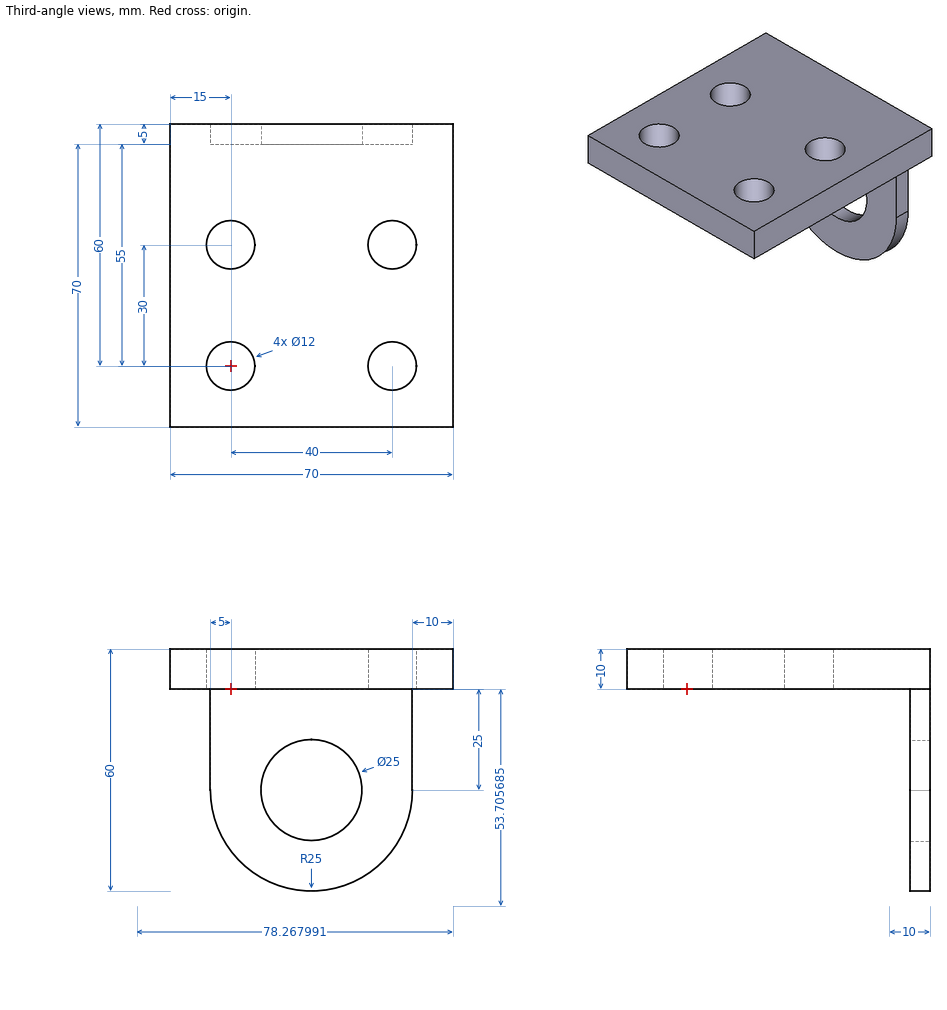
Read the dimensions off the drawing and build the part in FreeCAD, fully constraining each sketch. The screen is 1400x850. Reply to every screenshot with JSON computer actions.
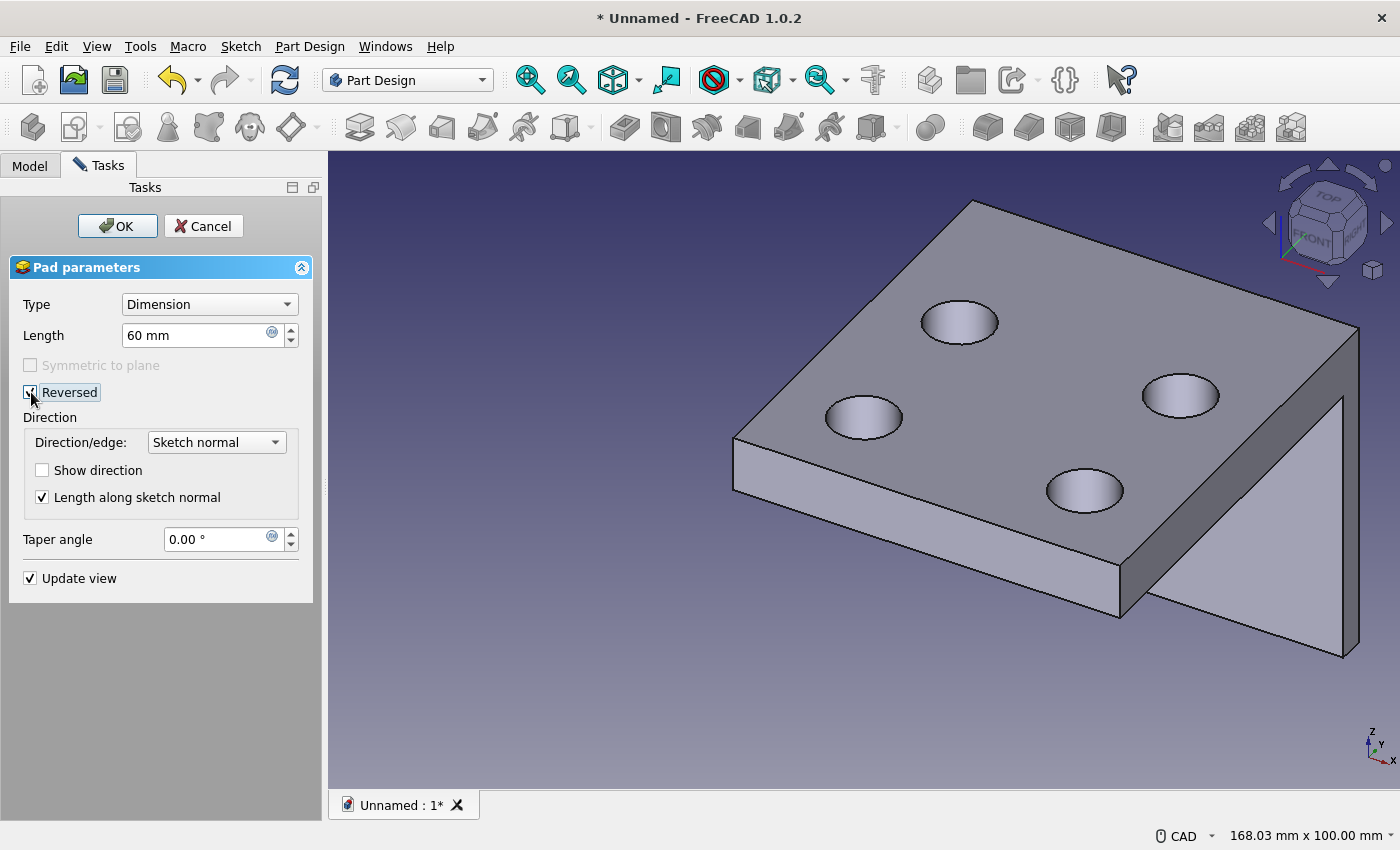
{"action": "left_click", "coordinate": [118, 226]}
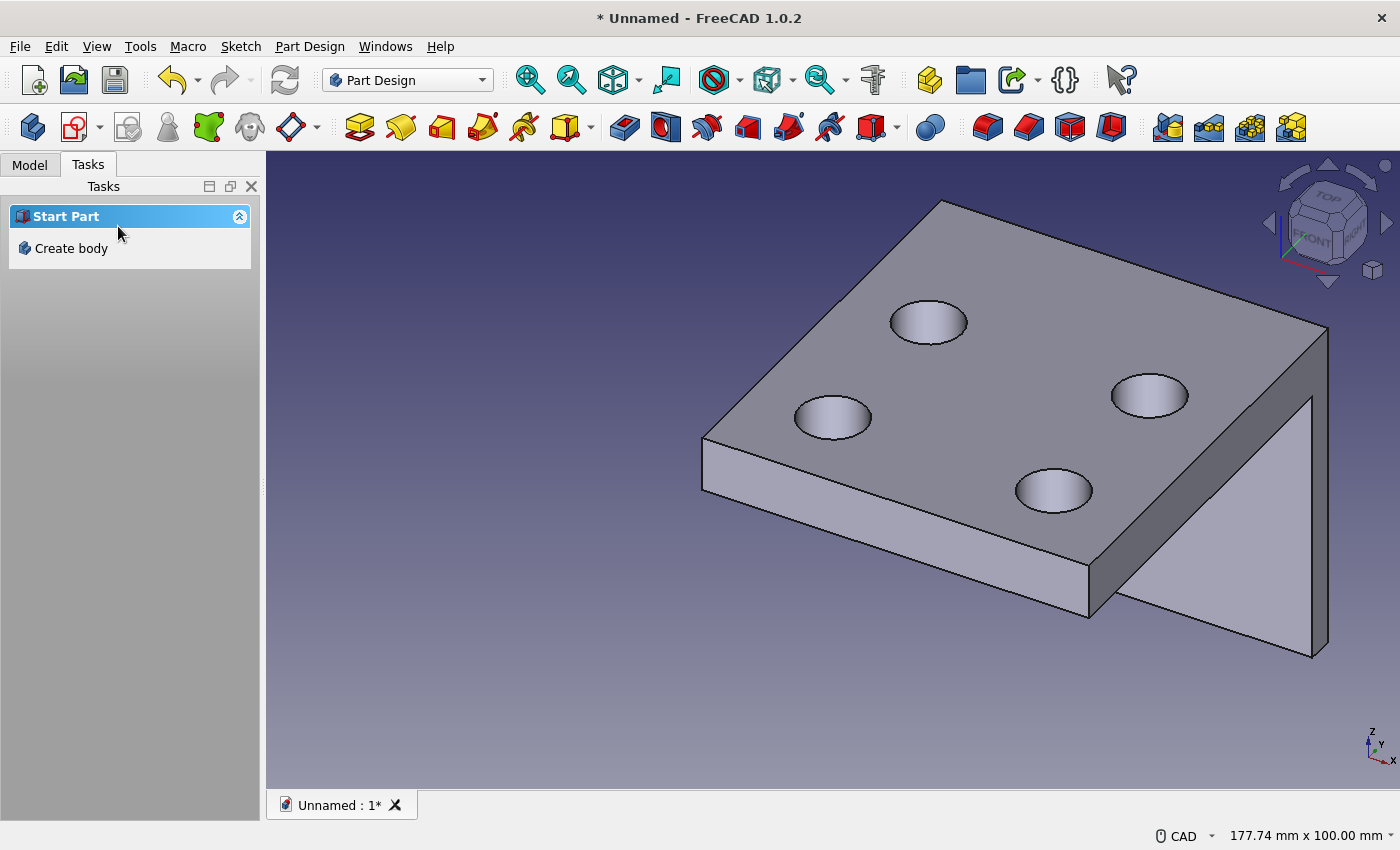
{"action": "left_click", "coordinate": [531, 80]}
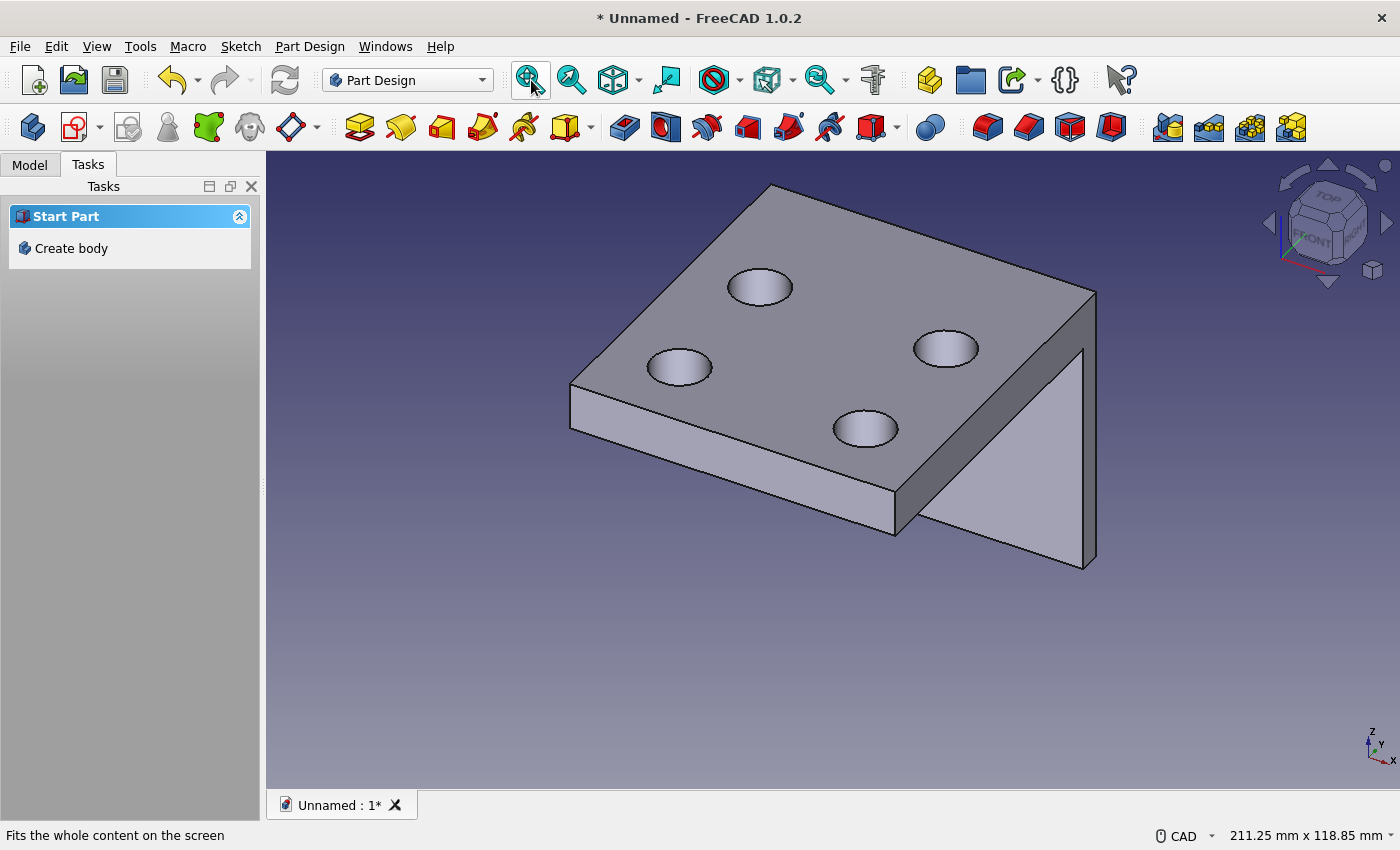
{"action": "key", "text": "4"}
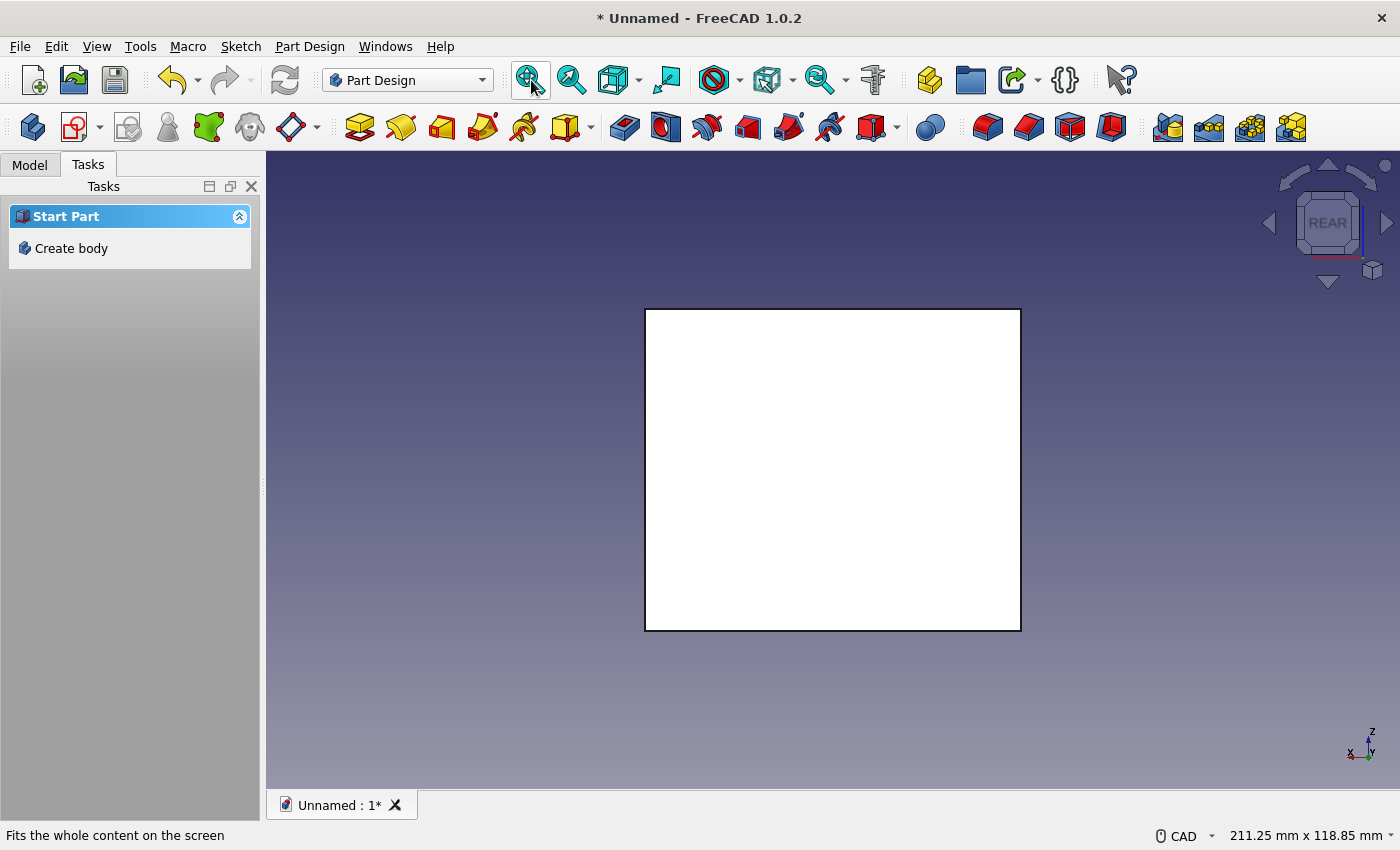
{"action": "left_click", "coordinate": [833, 469]}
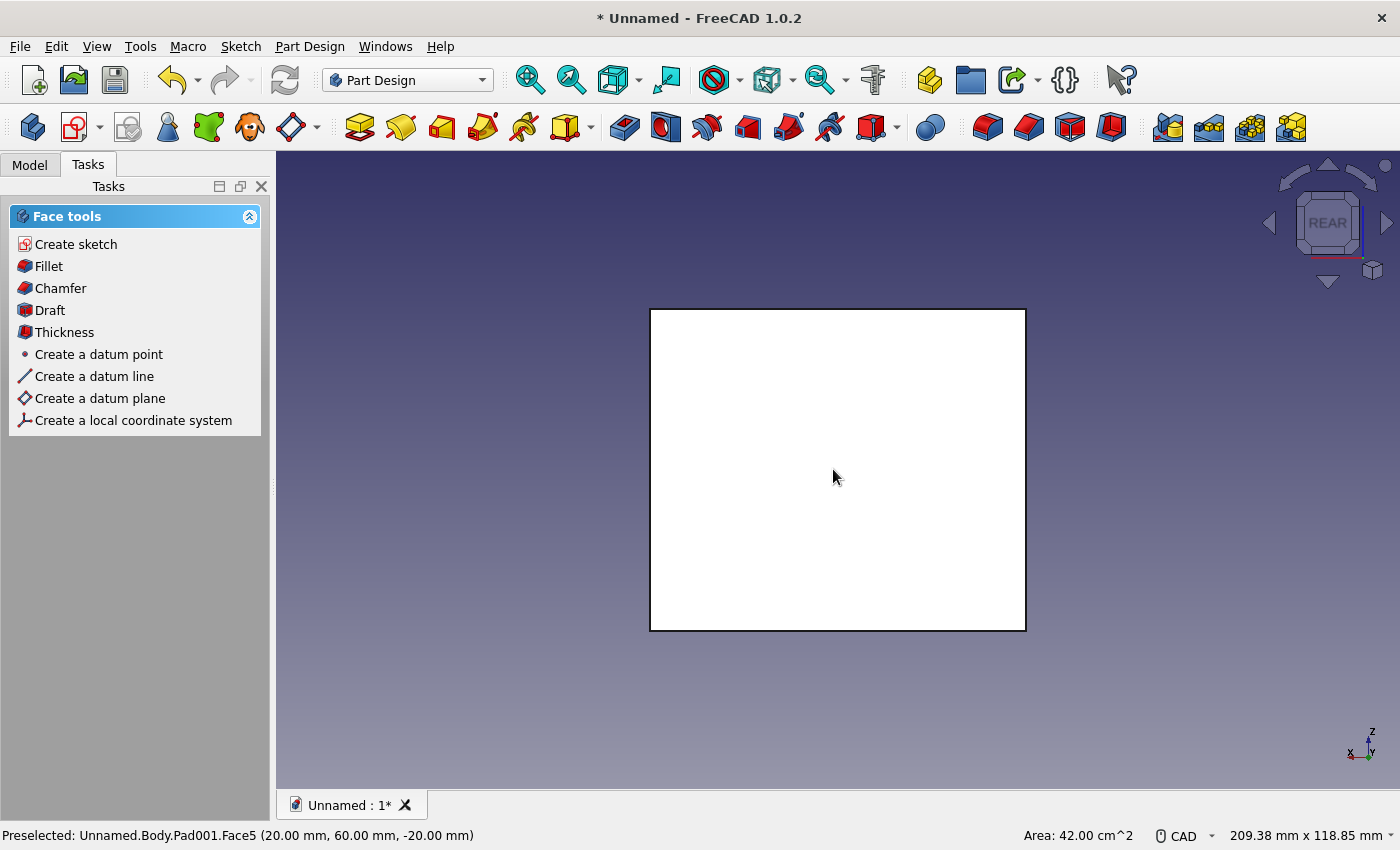
{"action": "left_click", "coordinate": [74, 128]}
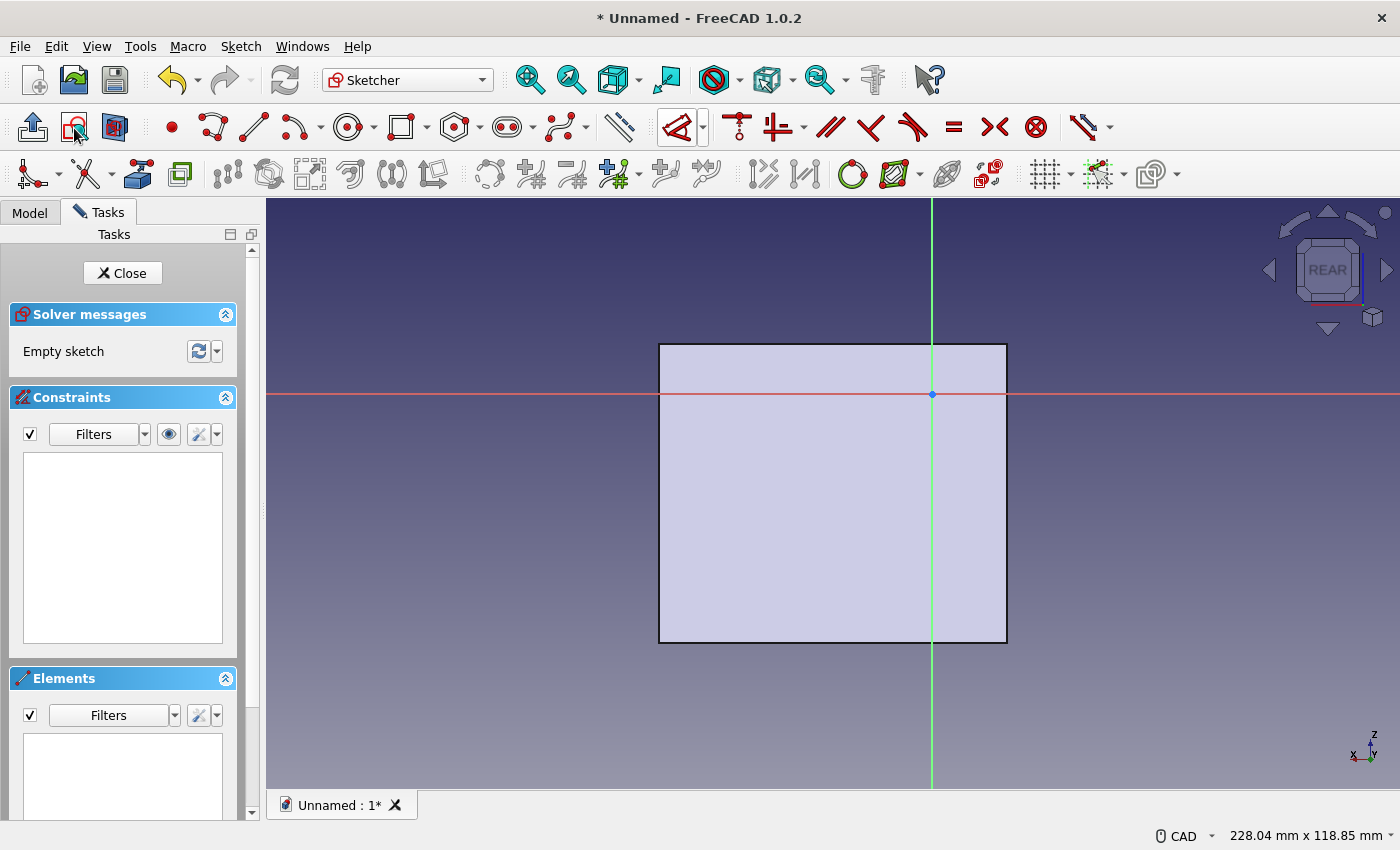
{"action": "scroll", "coordinate": [1035, 597], "scroll_direction": "up", "scroll_amount": 2}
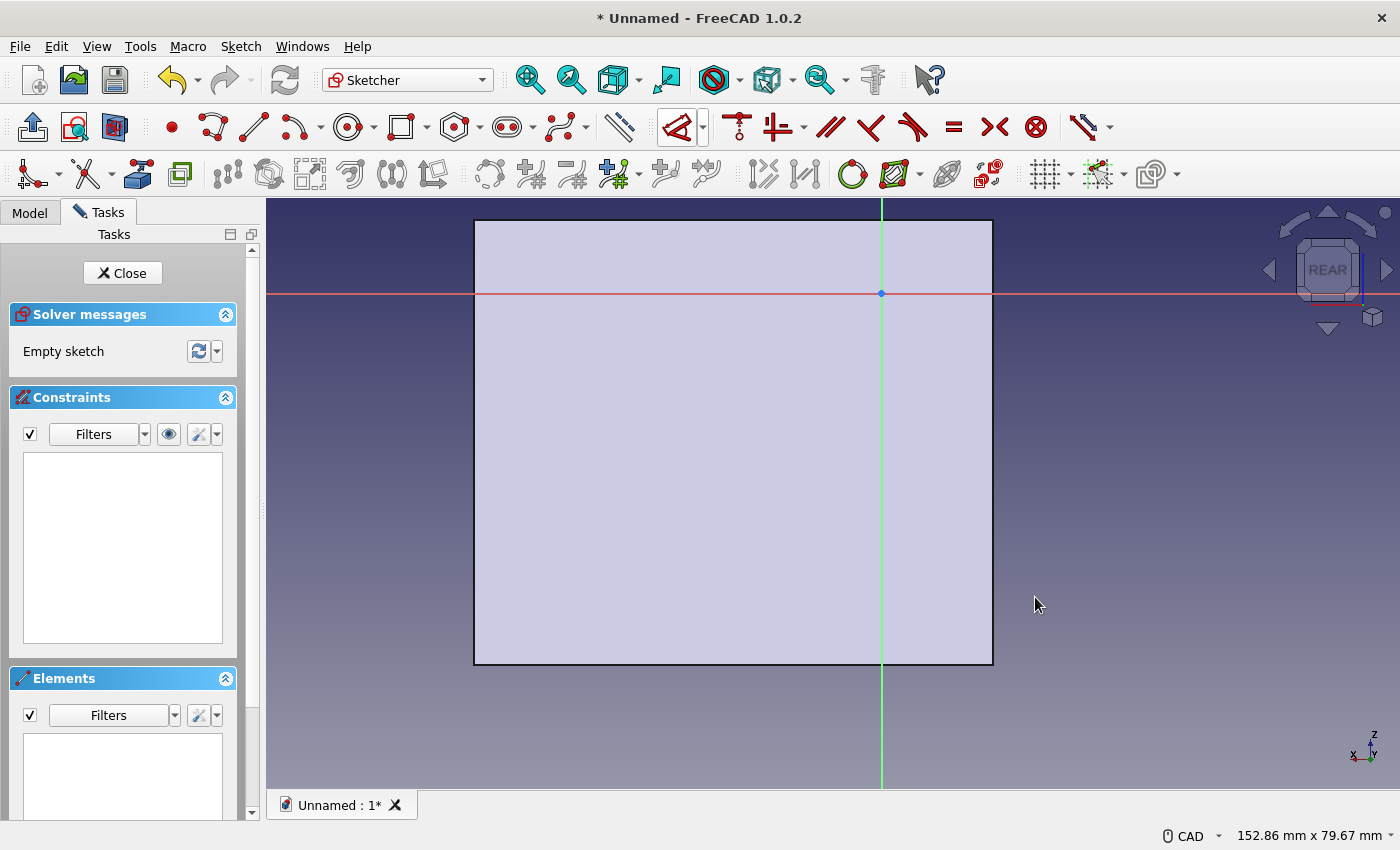
{"action": "key", "text": "g m"}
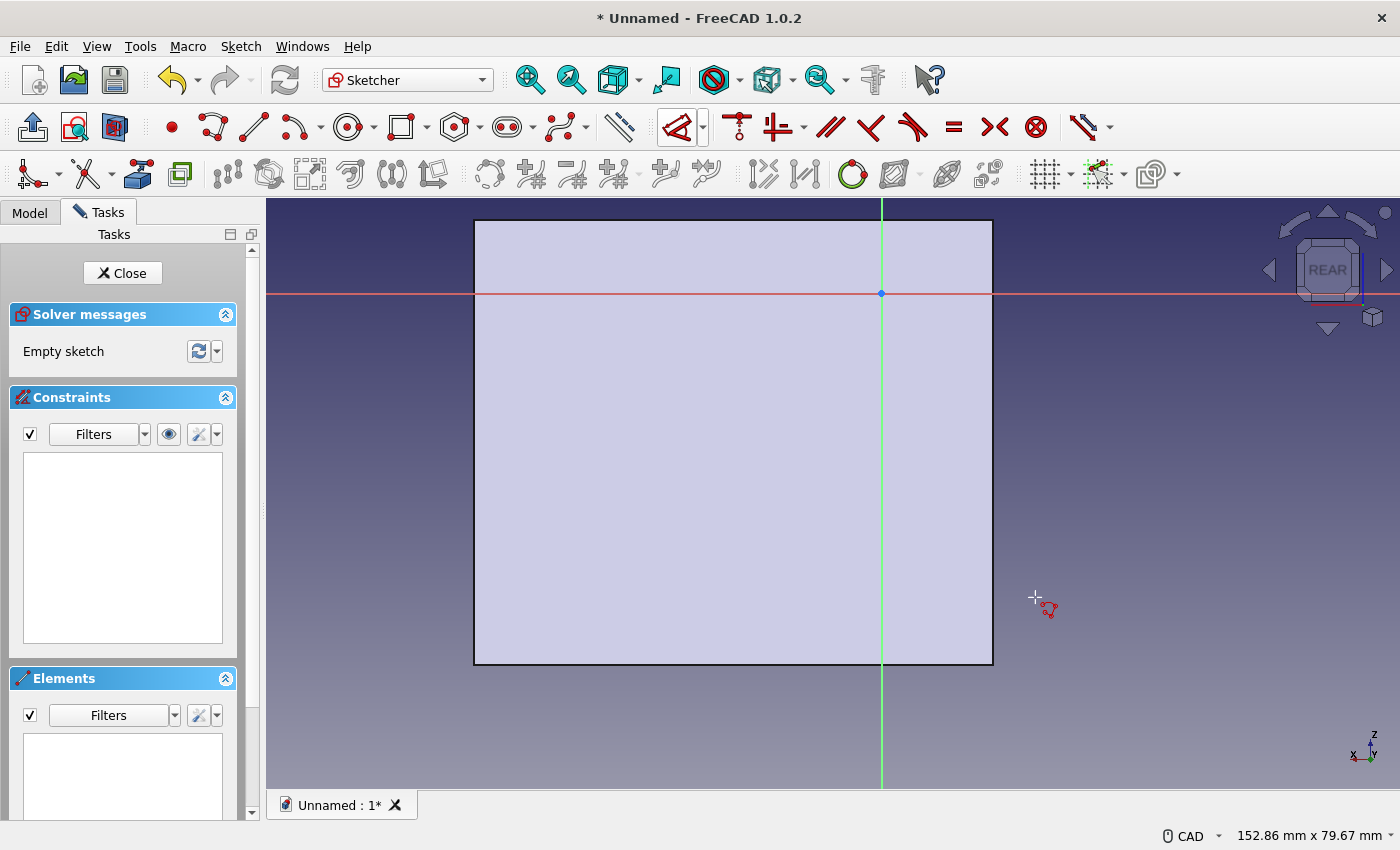
{"action": "left_click", "coordinate": [548, 479]}
{"action": "left_click", "coordinate": [548, 294]}
{"action": "left_click", "coordinate": [474, 303]}
{"action": "left_click", "coordinate": [474, 692]}
{"action": "left_click", "coordinate": [1054, 692]}
{"action": "left_click", "coordinate": [1054, 294]}
{"action": "left_click", "coordinate": [919, 303]}
{"action": "left_click", "coordinate": [919, 479]}
{"action": "right_click", "coordinate": [919, 479]}